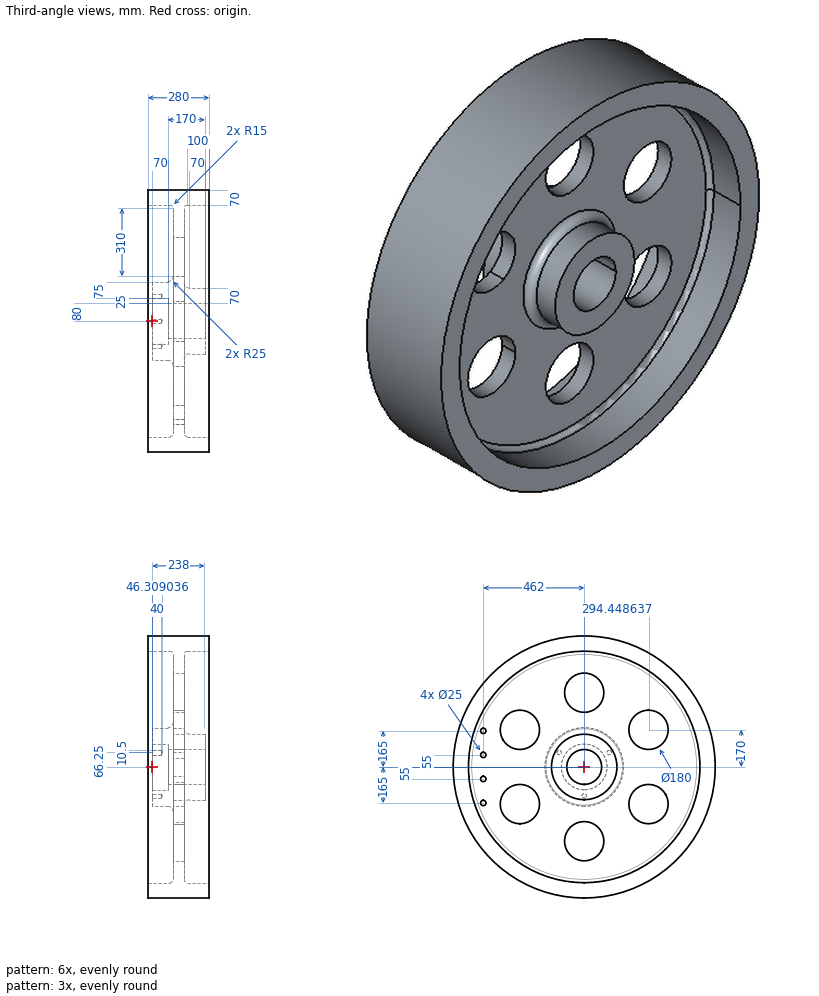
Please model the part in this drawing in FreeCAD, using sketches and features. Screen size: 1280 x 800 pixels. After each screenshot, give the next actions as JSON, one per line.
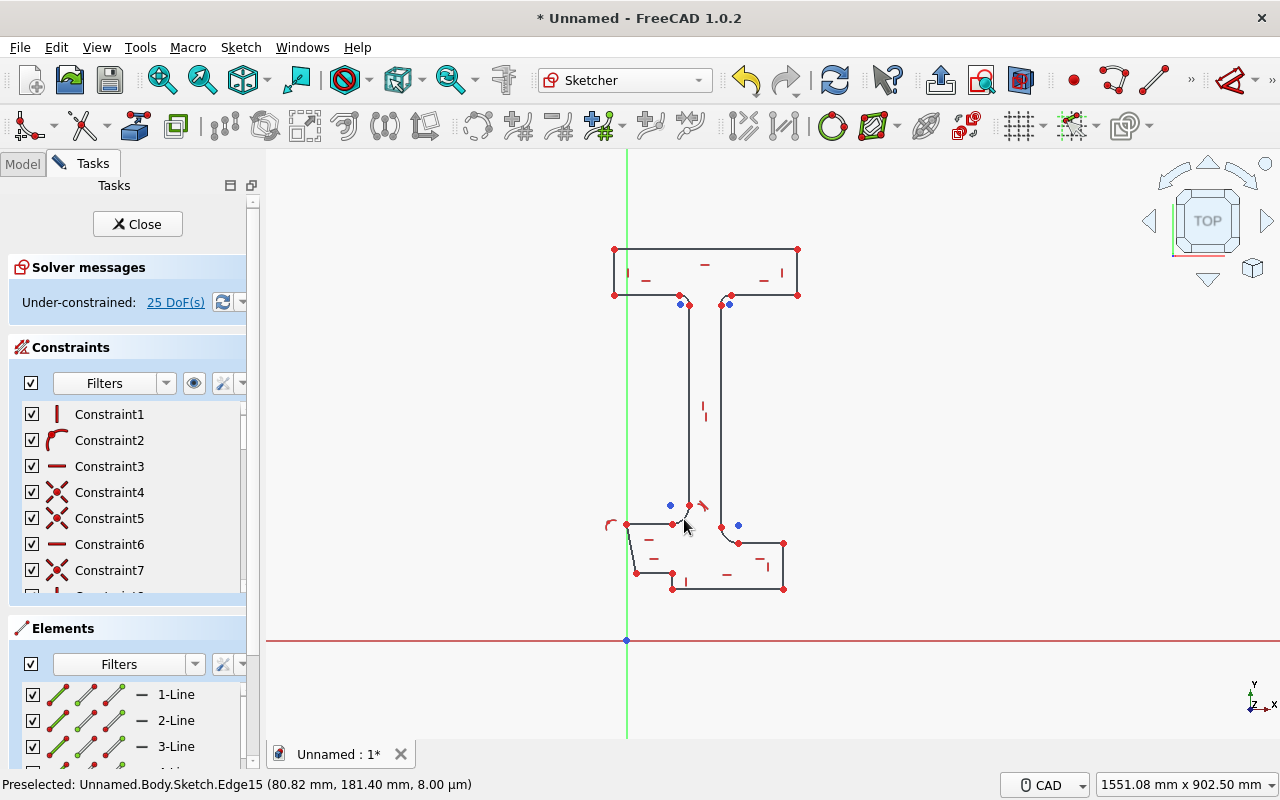
{"action": "left_click", "coordinate": [689, 365]}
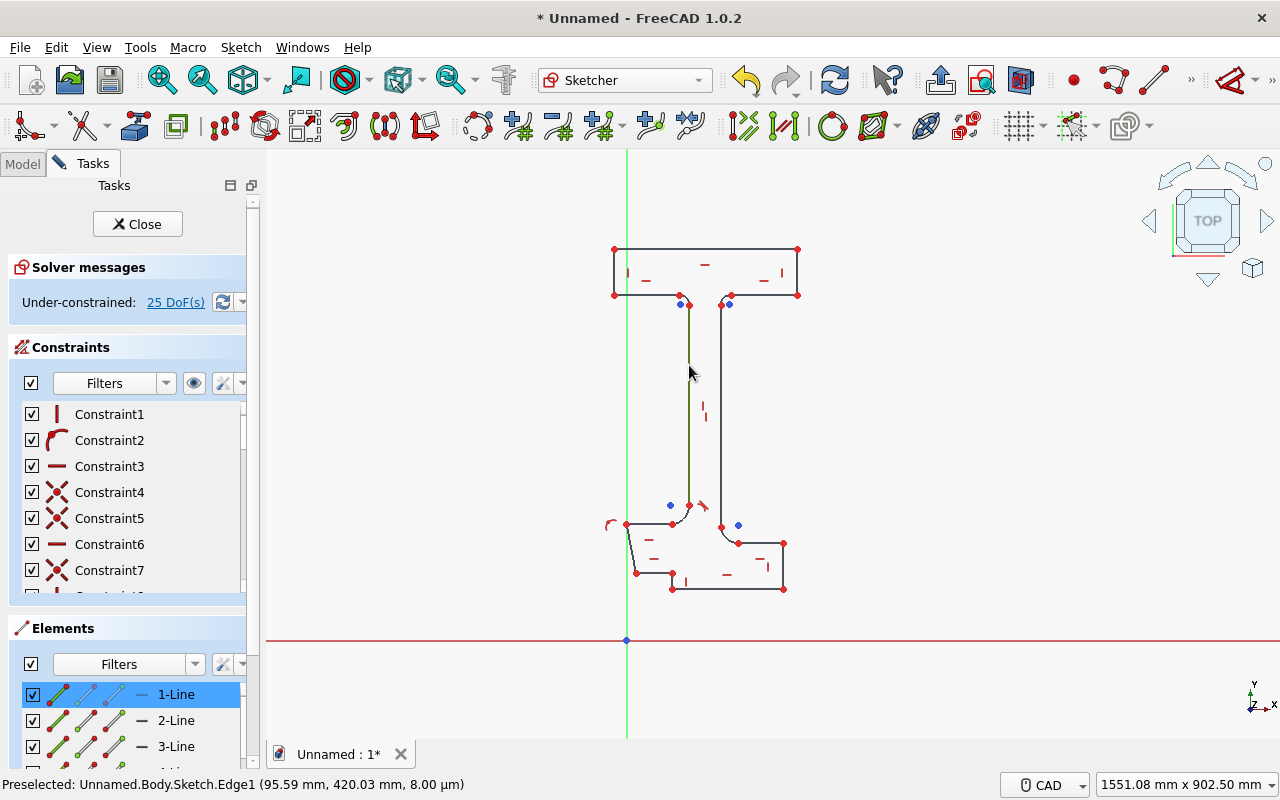
{"action": "scroll", "coordinate": [687, 298], "scroll_direction": "up", "scroll_amount": 3}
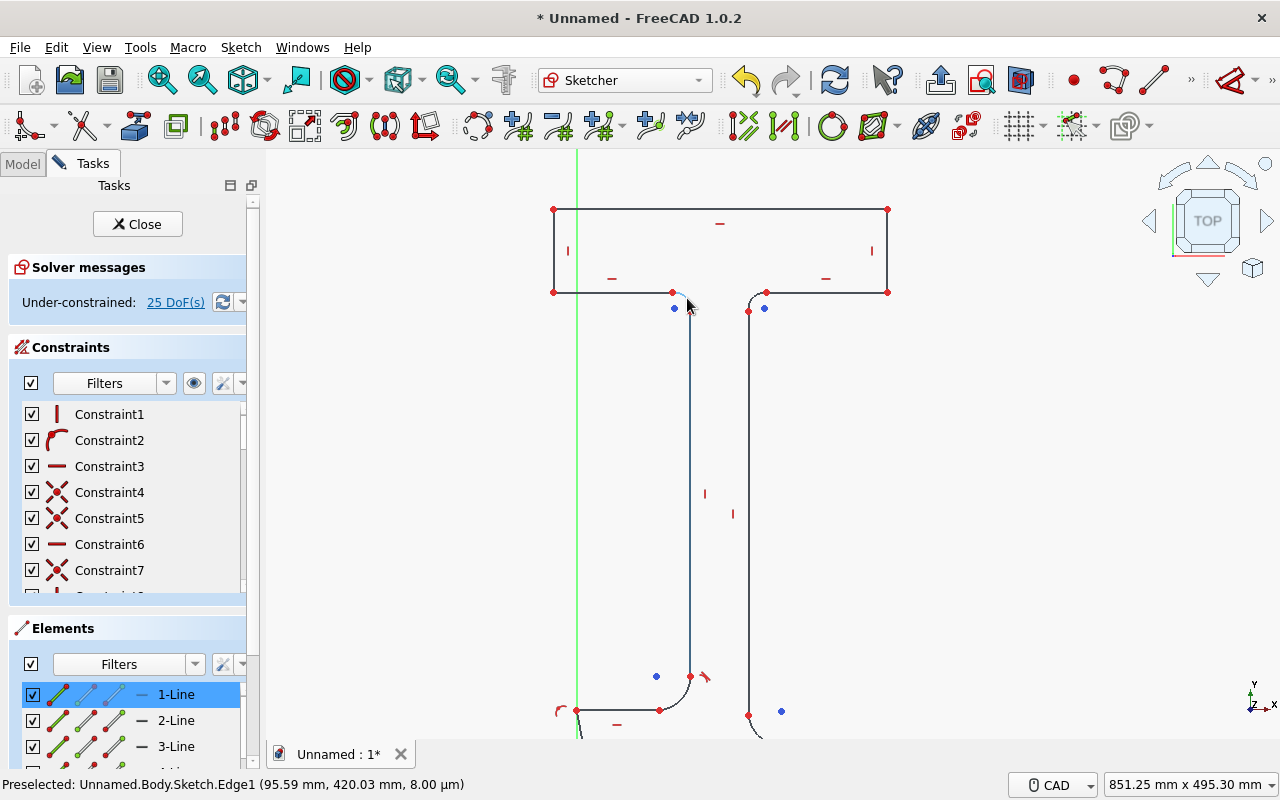
{"action": "left_click", "coordinate": [686, 297]}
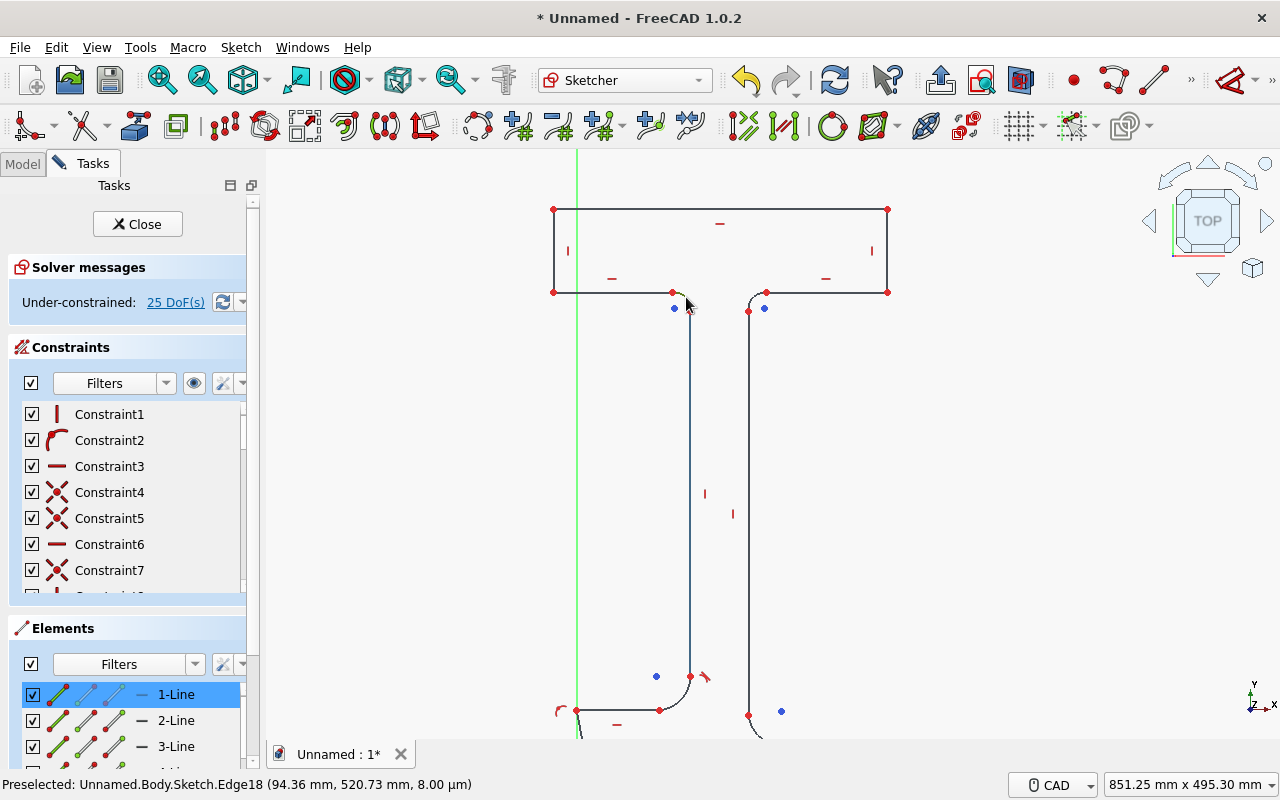
{"action": "key", "text": "t"}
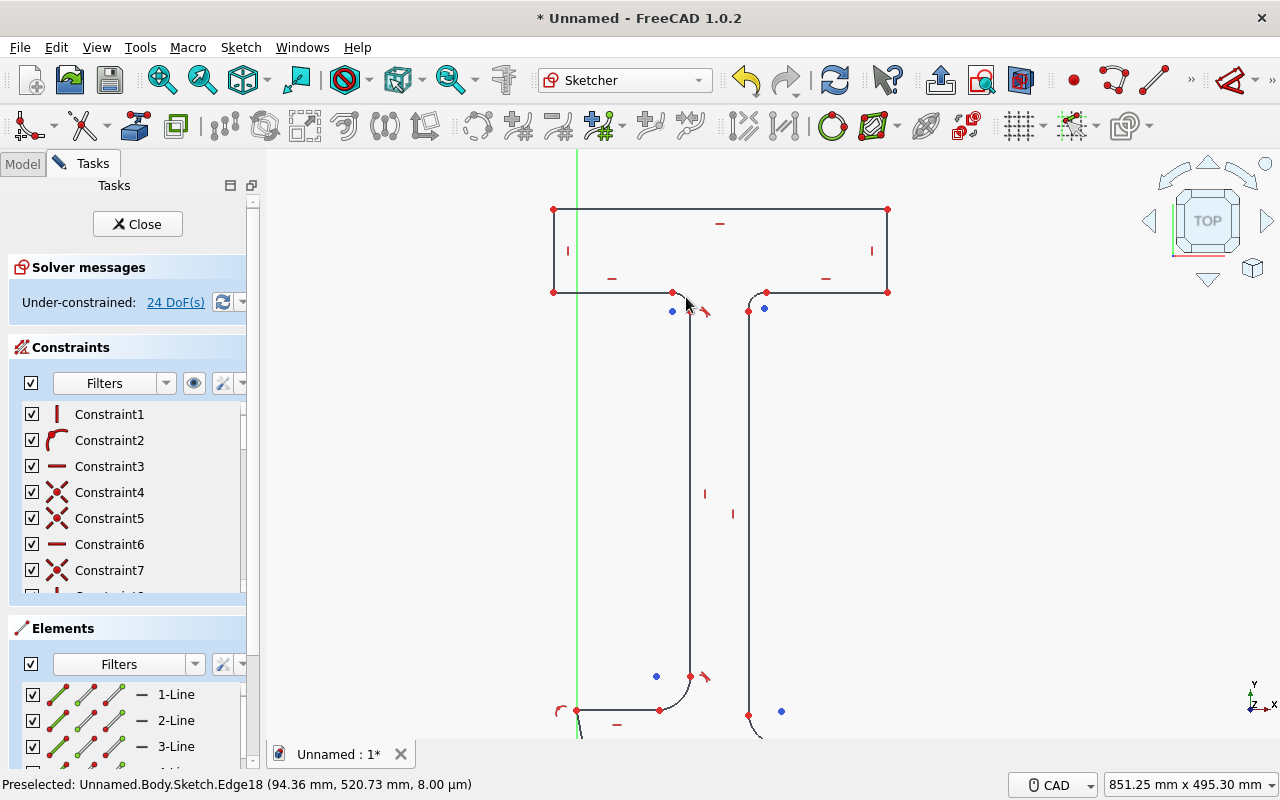
{"action": "left_click", "coordinate": [634, 710]}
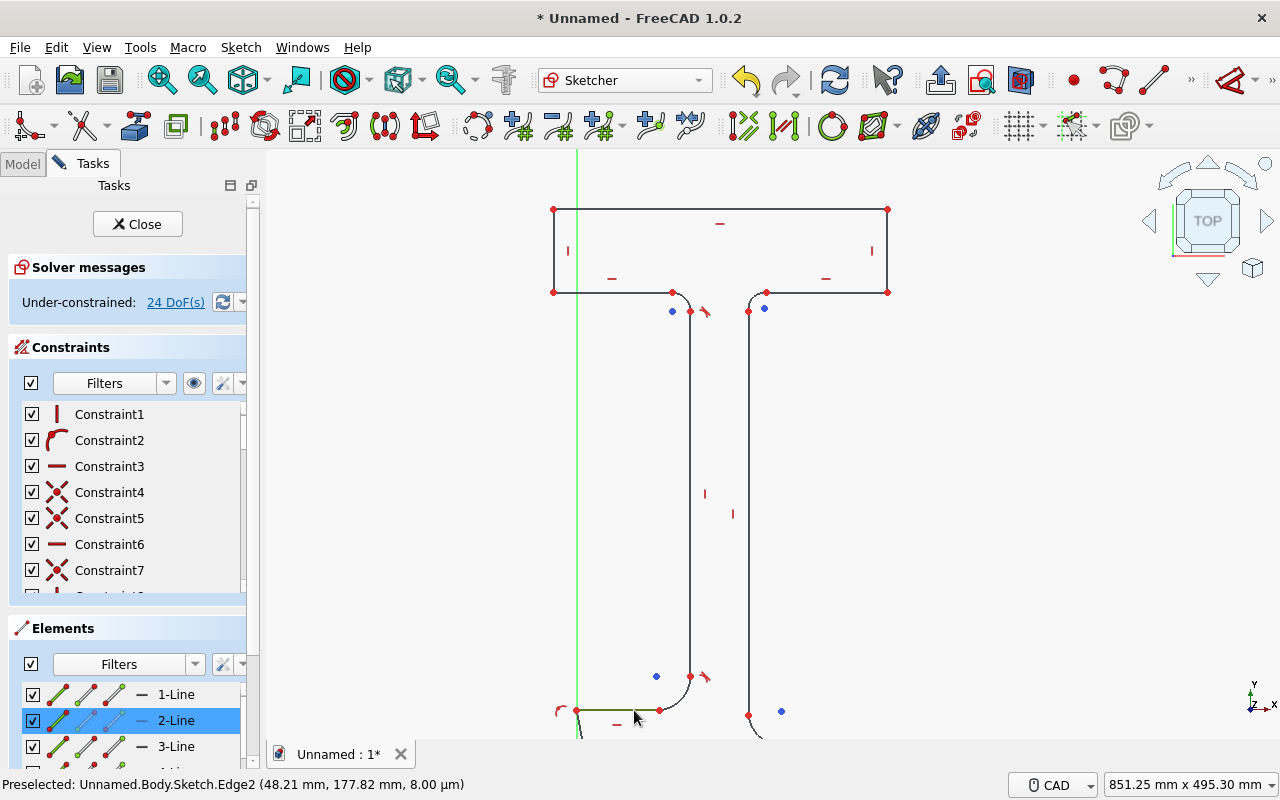
{"action": "left_click", "coordinate": [674, 706]}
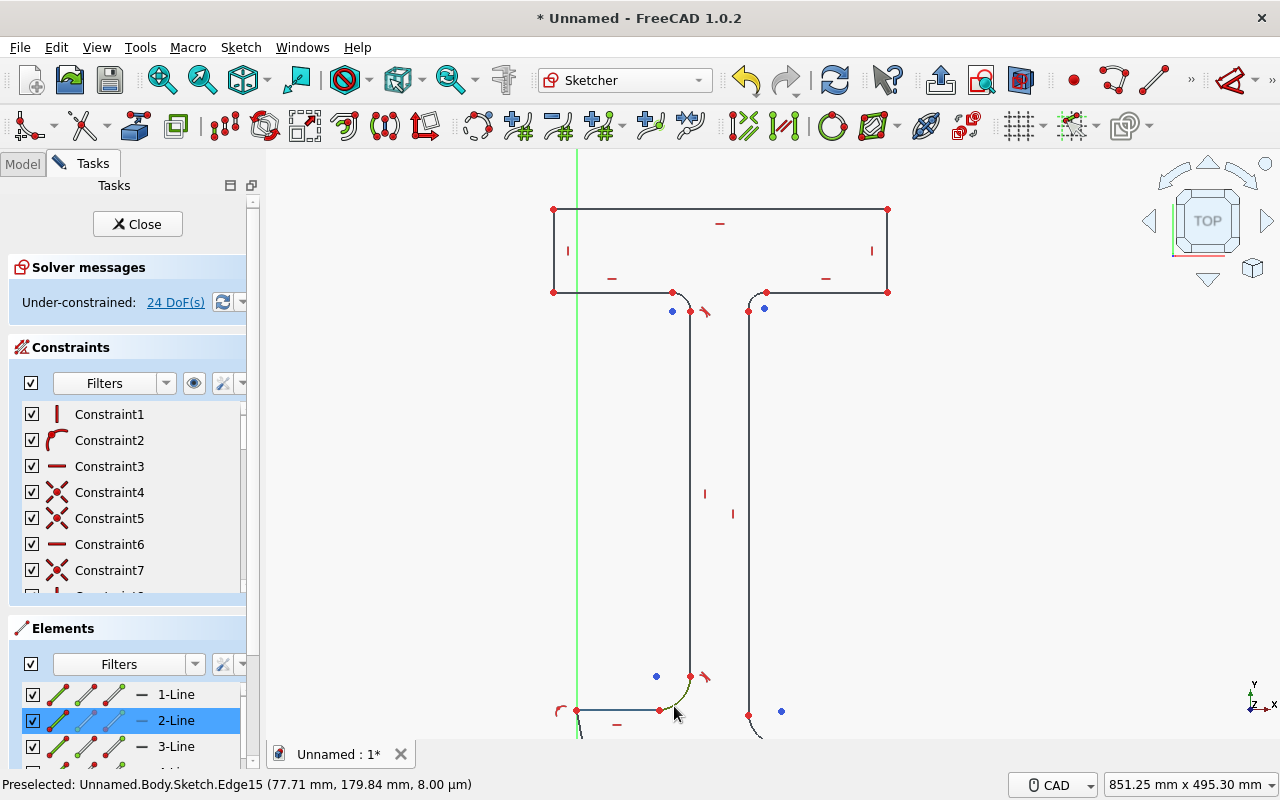
{"action": "key", "text": "t"}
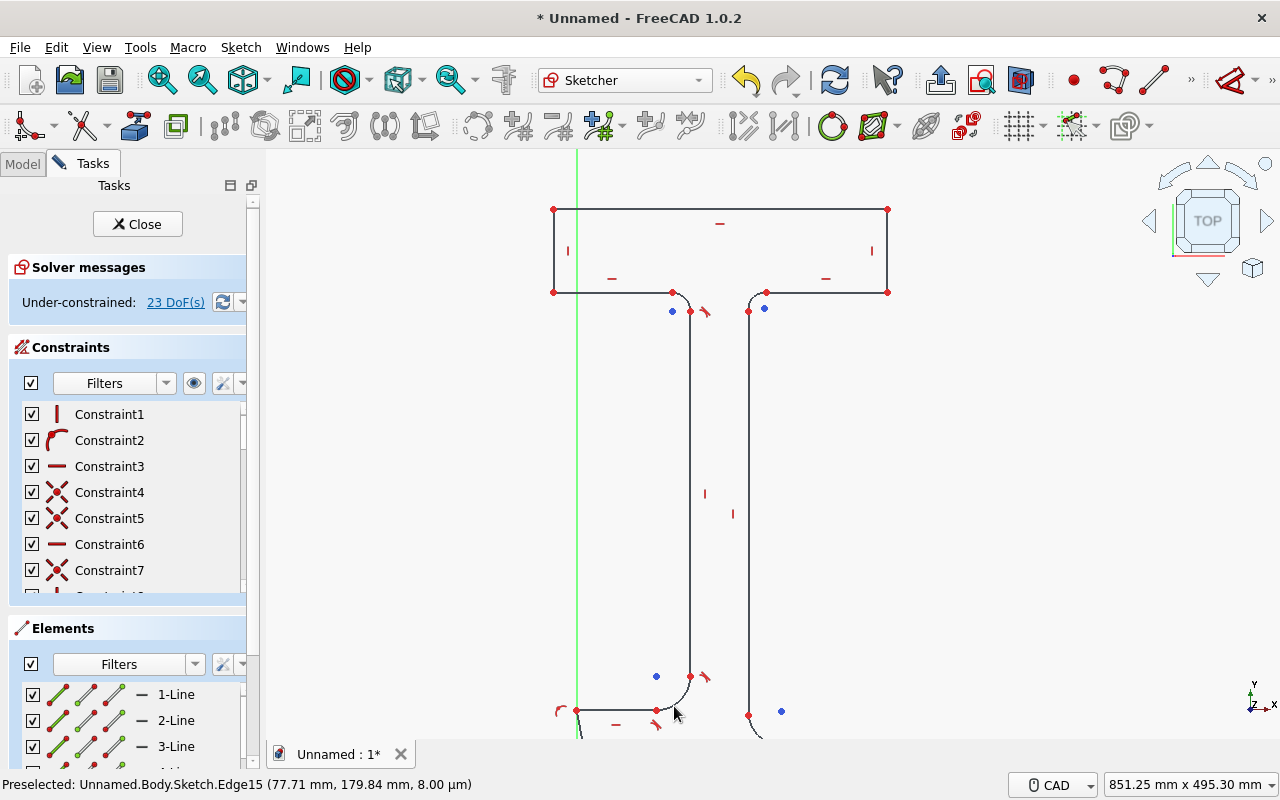
{"action": "scroll", "coordinate": [686, 297], "scroll_direction": "down", "scroll_amount": 3}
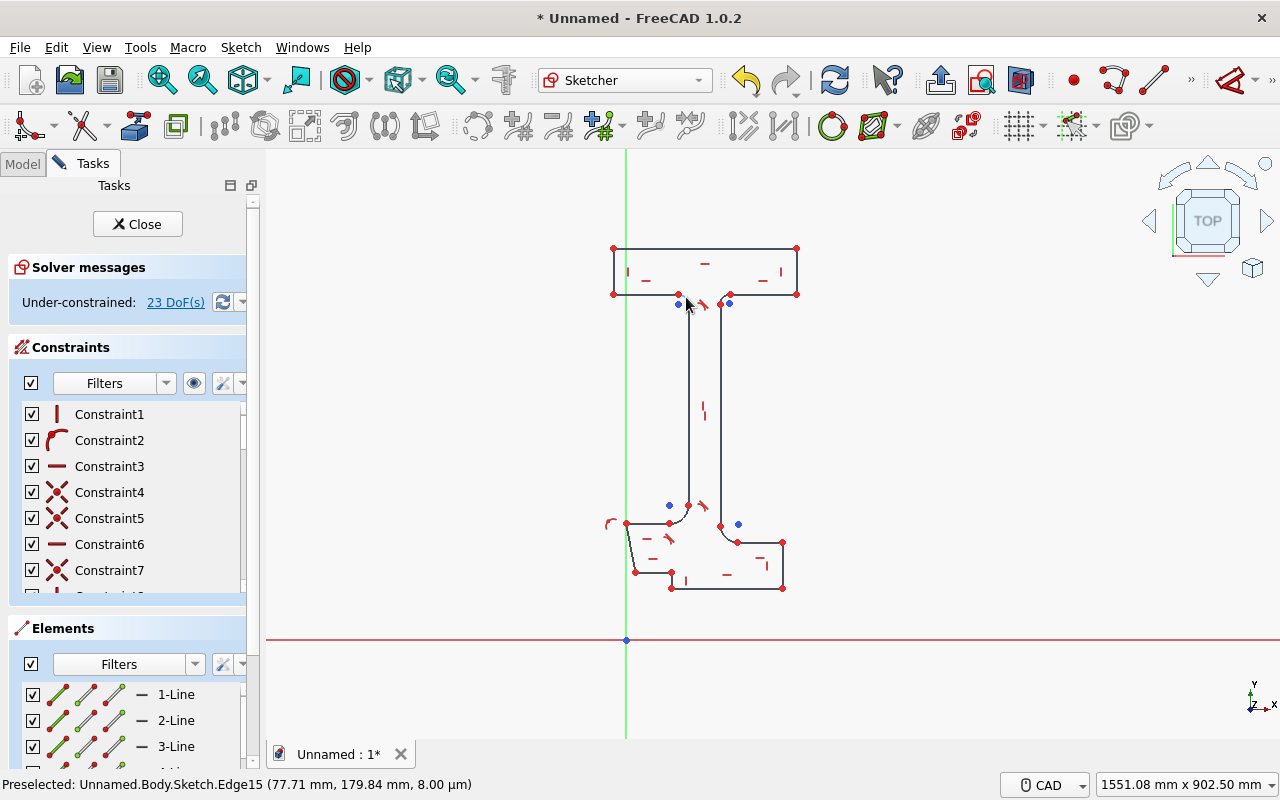
{"action": "left_click", "coordinate": [769, 543]}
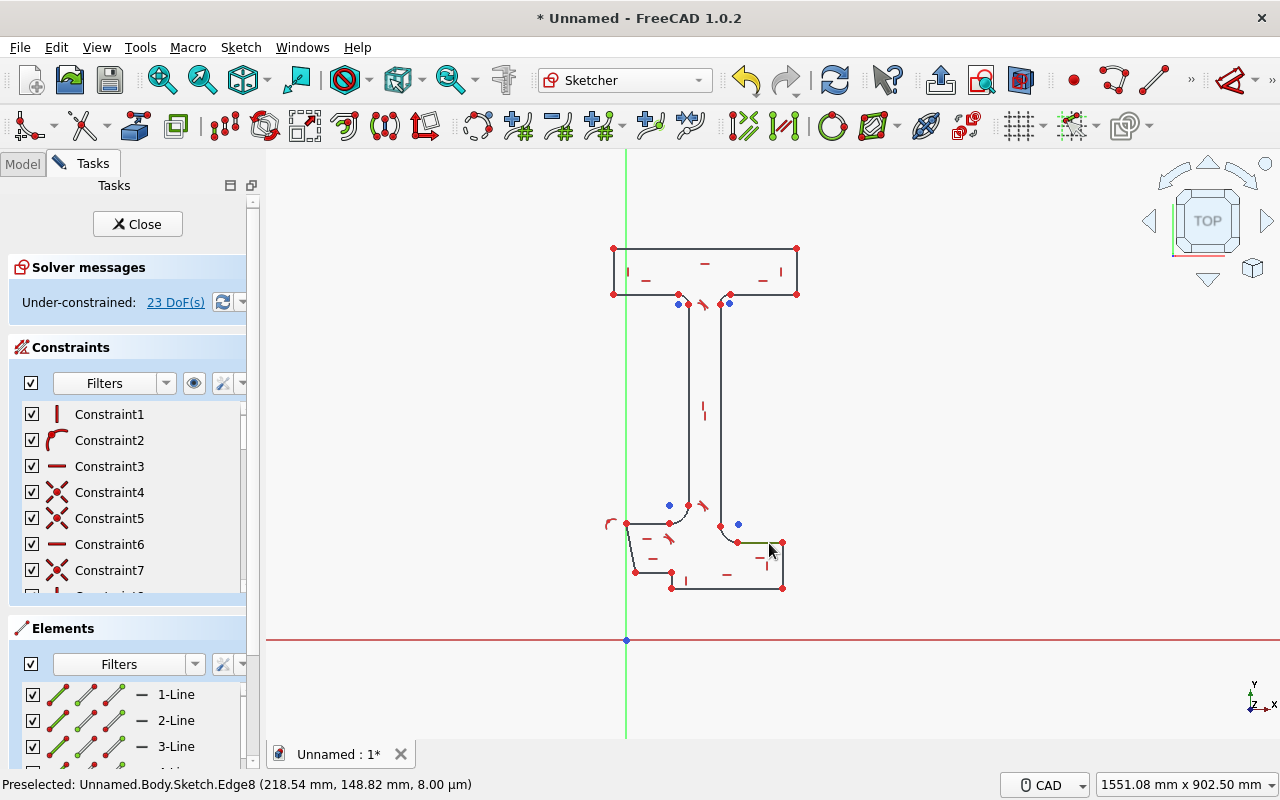
{"action": "left_click", "coordinate": [726, 538]}